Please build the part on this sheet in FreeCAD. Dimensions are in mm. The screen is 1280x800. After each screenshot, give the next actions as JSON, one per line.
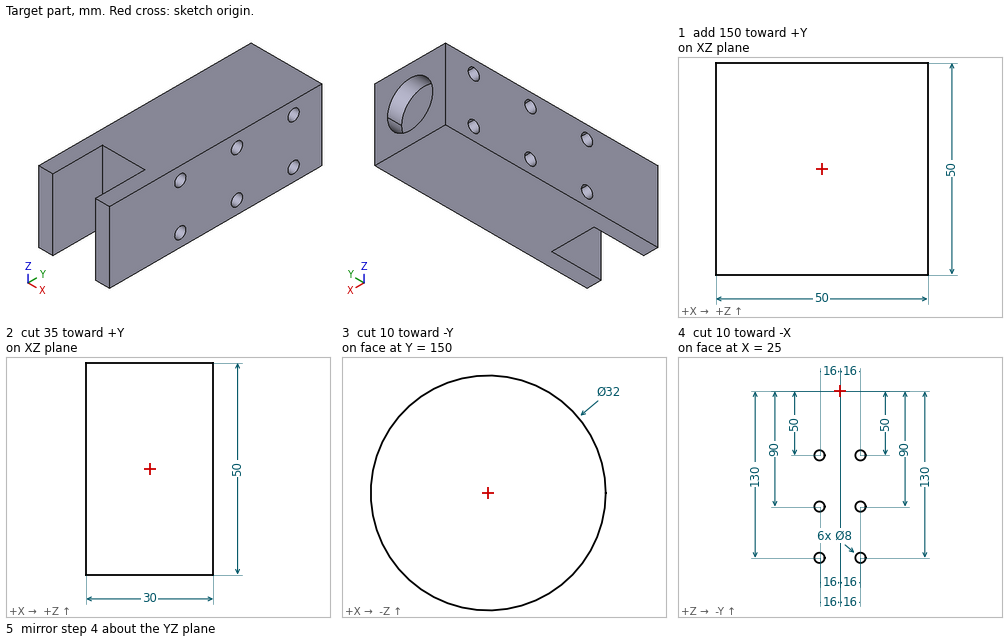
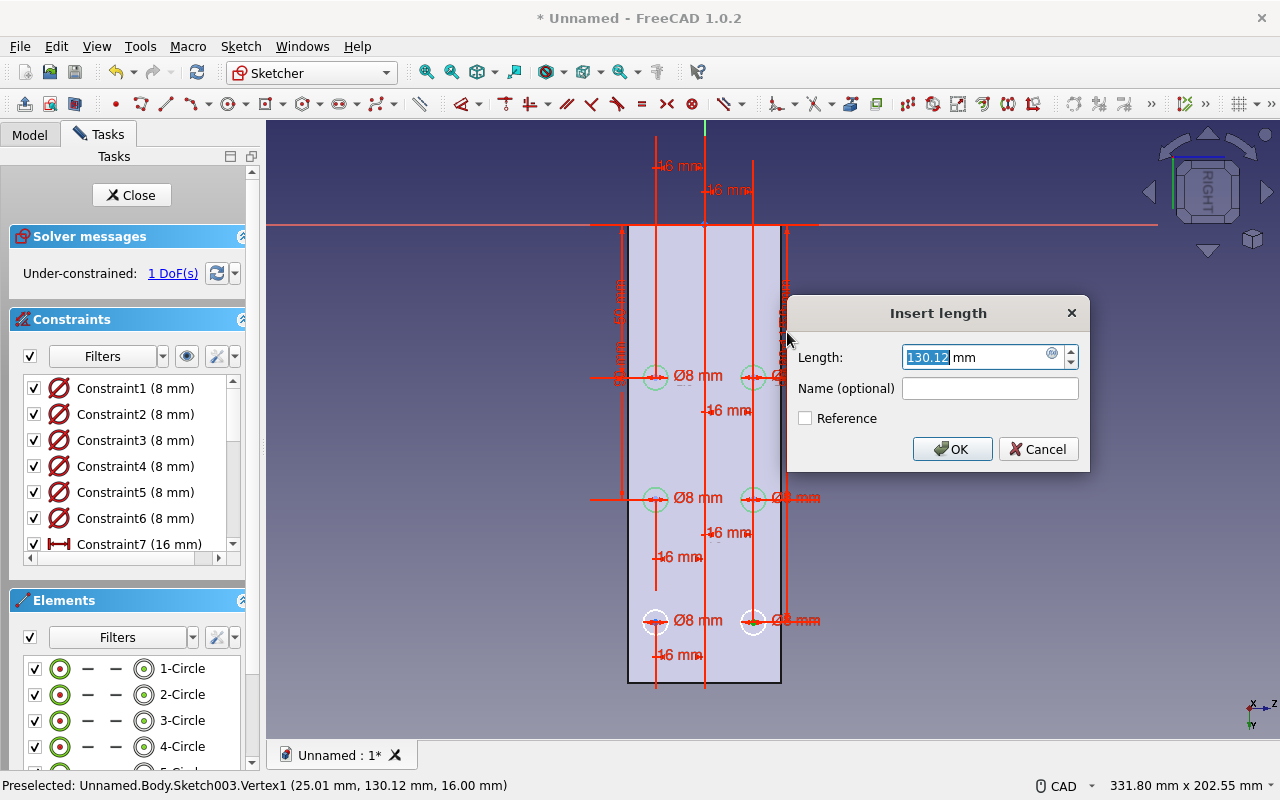
{"action": "type", "text": "130"}
{"action": "key", "text": "Return"}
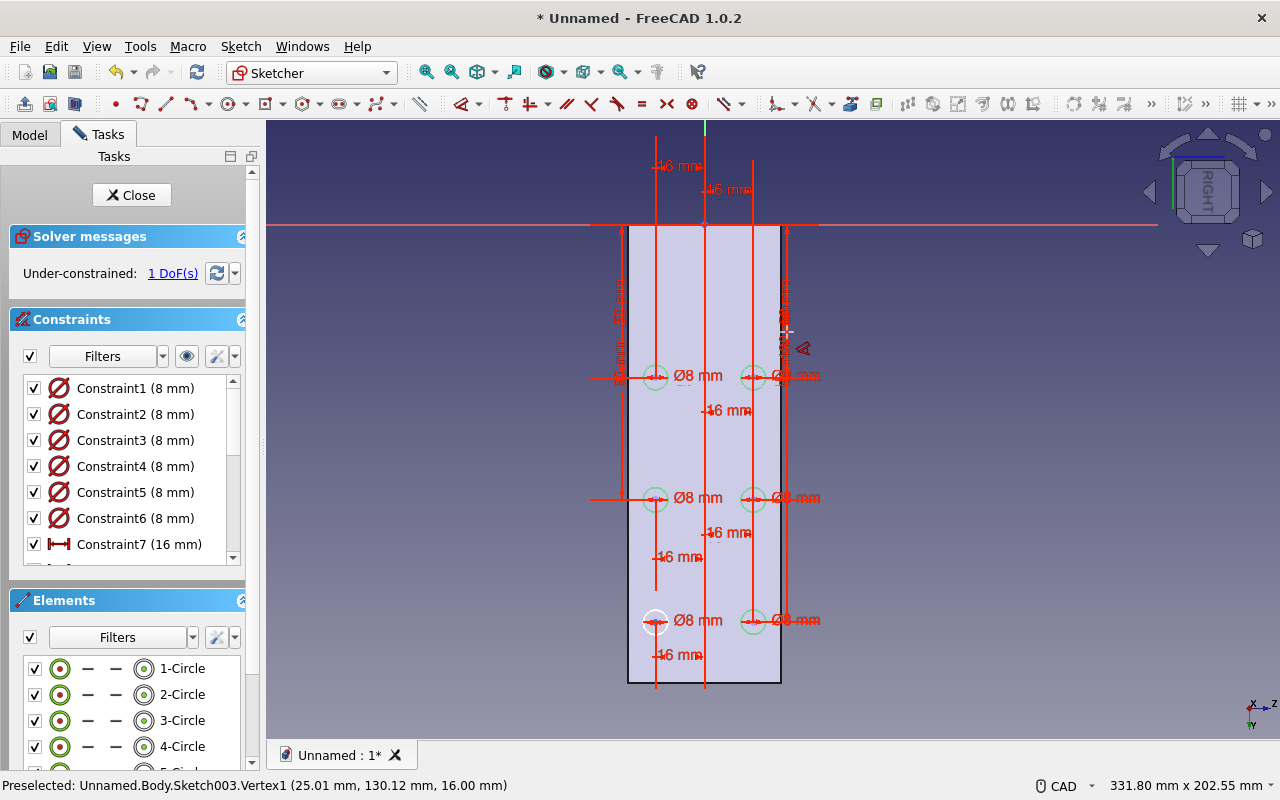
{"action": "left_click", "coordinate": [656, 622]}
{"action": "left_click", "coordinate": [622, 424]}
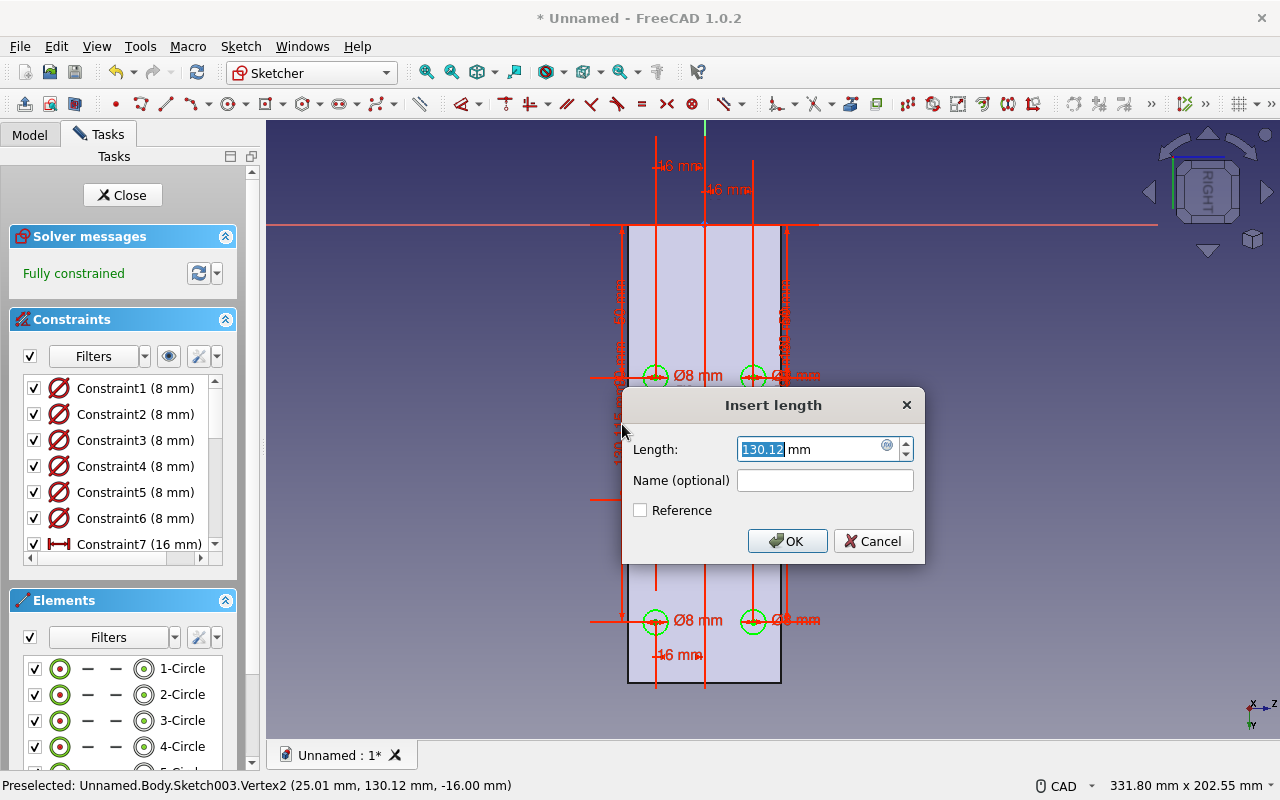
{"action": "type", "text": "130"}
{"action": "key", "text": "Return"}
{"action": "key", "text": "Escape"}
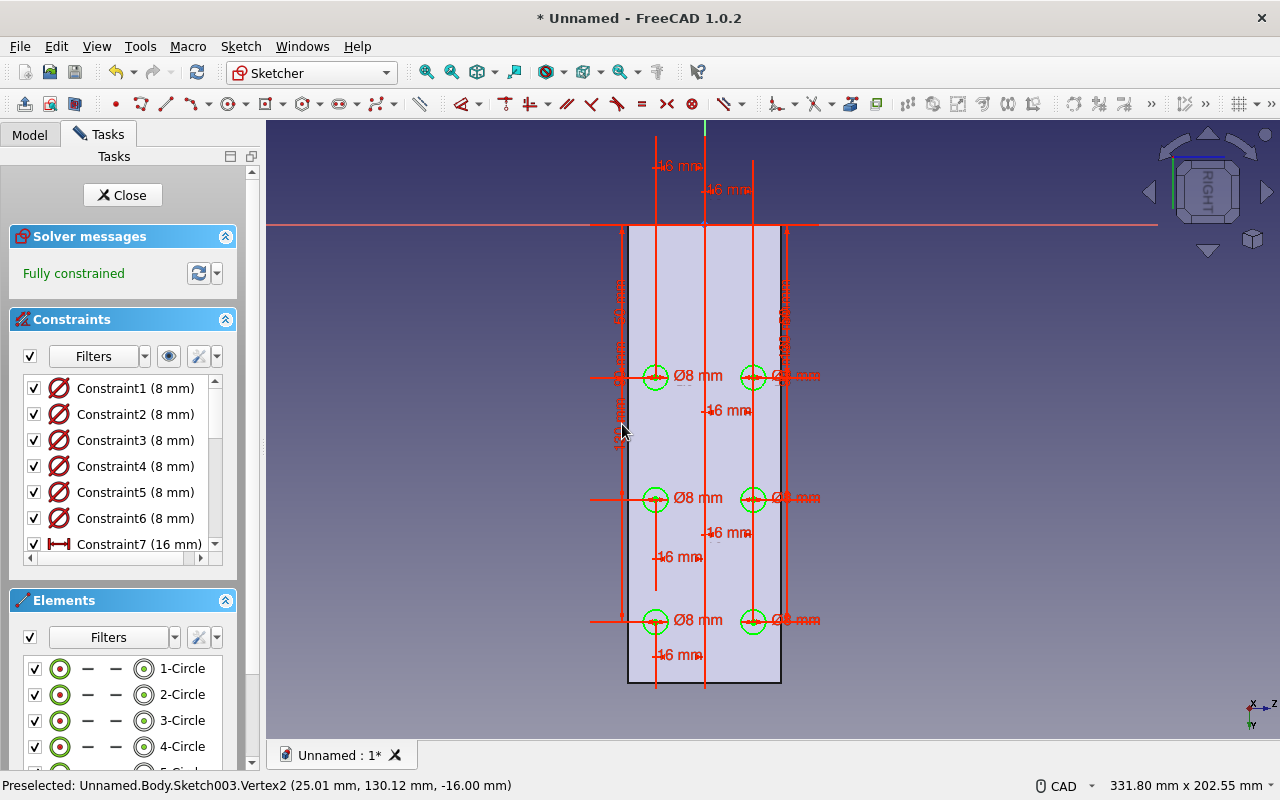
{"action": "left_click", "coordinate": [123, 195]}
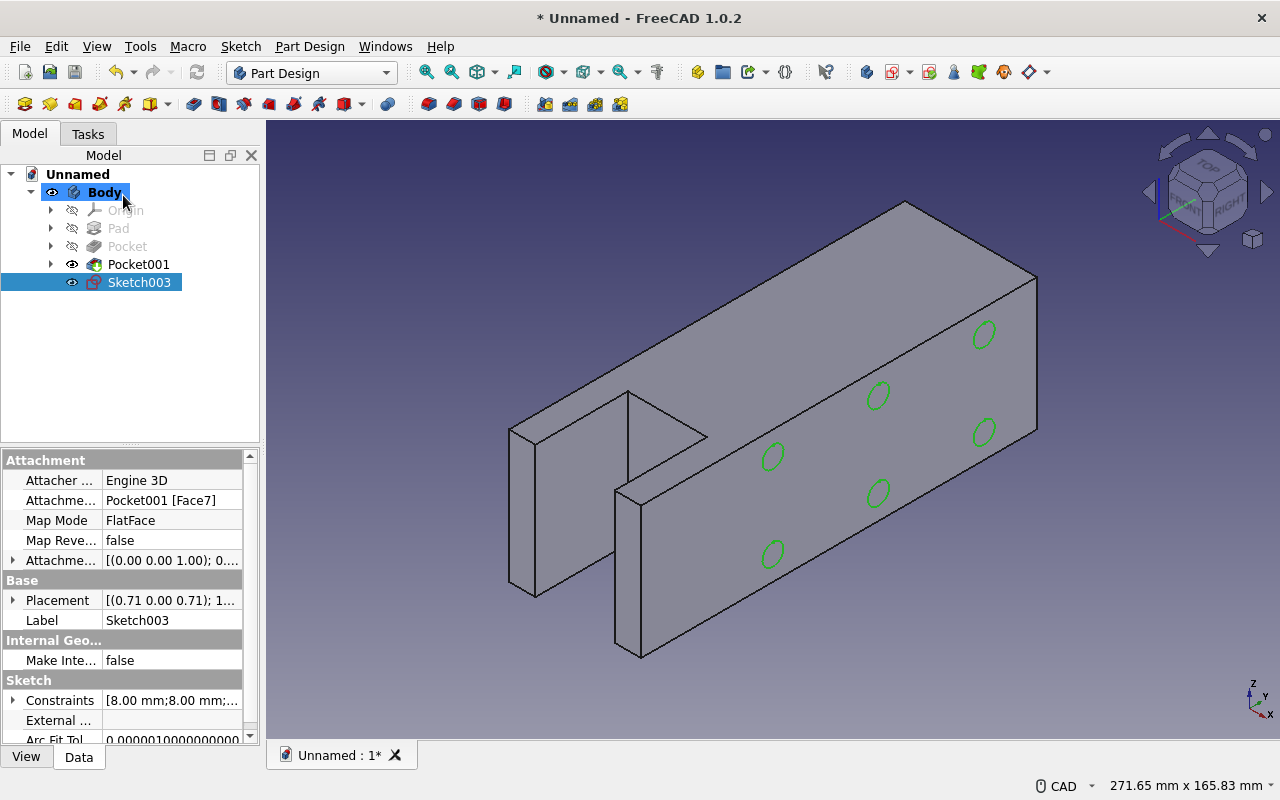
{"action": "left_click", "coordinate": [194, 104]}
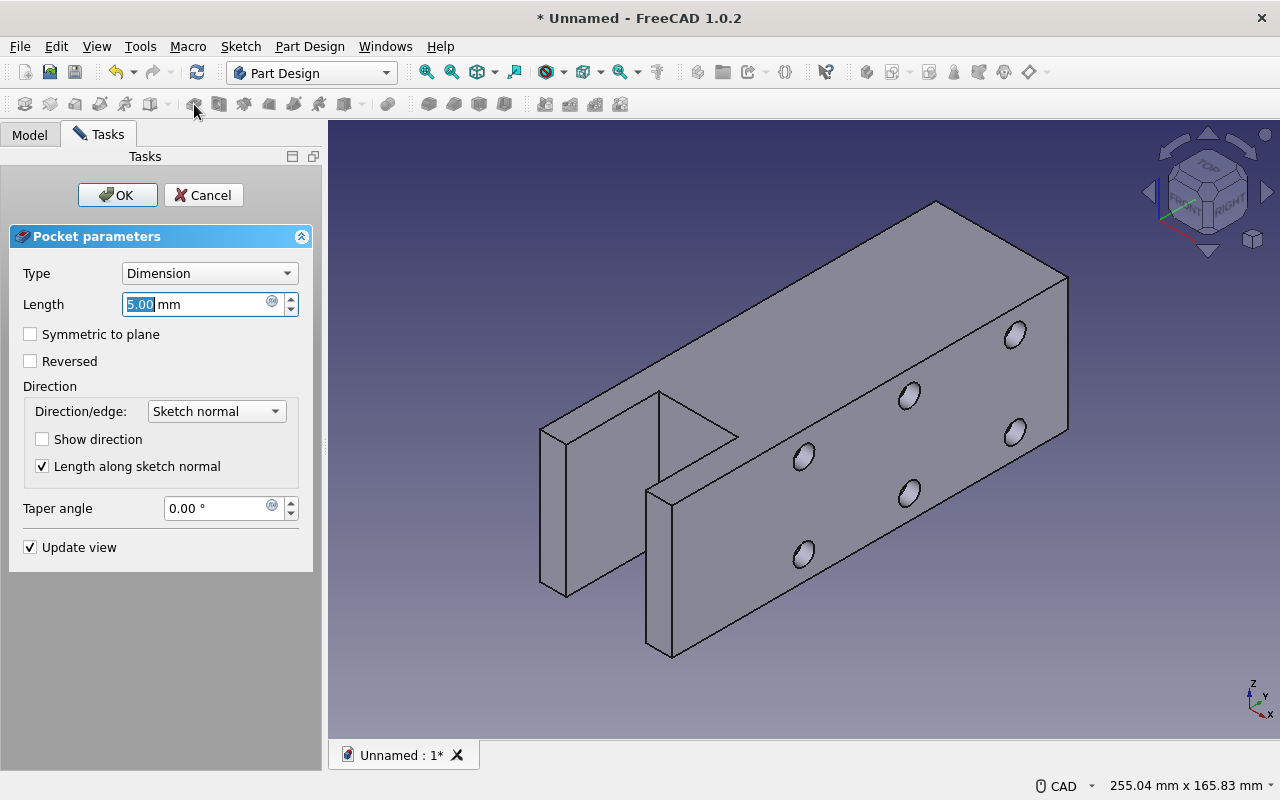
{"action": "type", "text": "10"}
{"action": "key", "text": "Tab"}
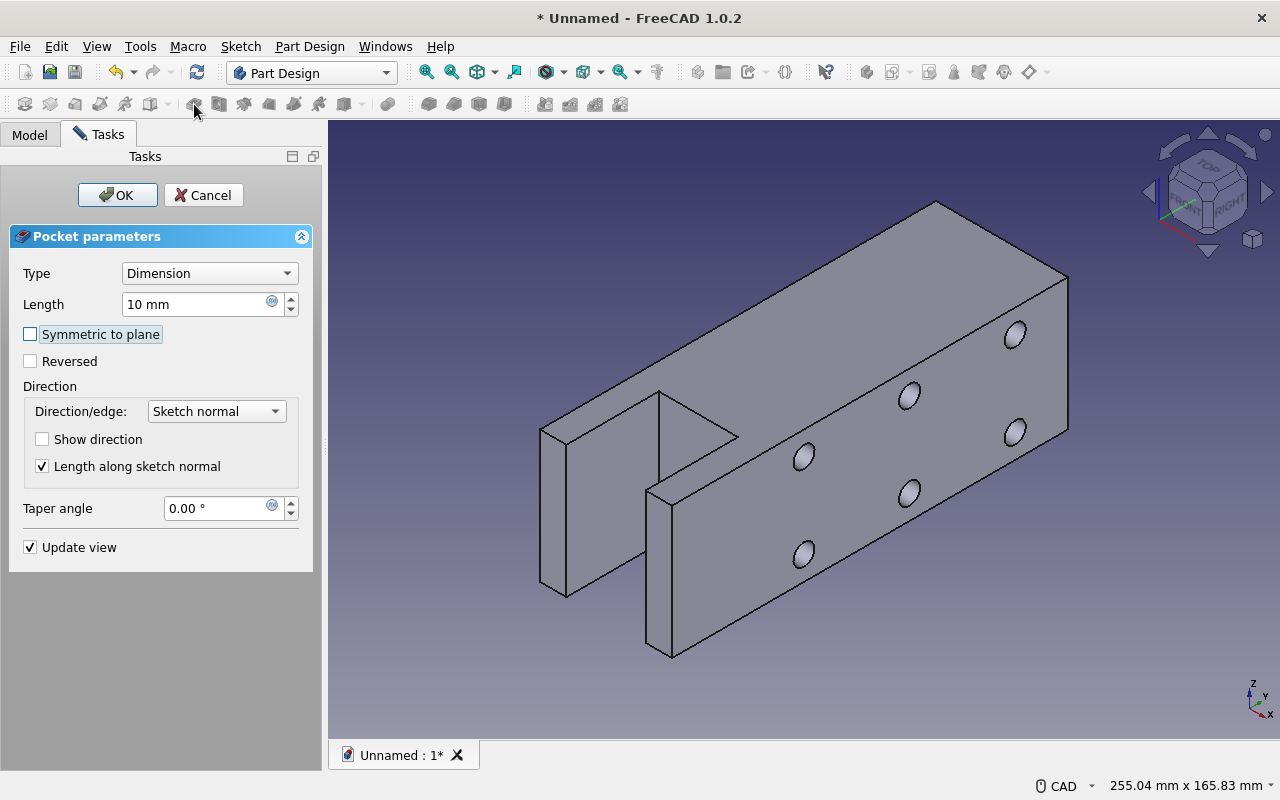
{"action": "left_click", "coordinate": [118, 195]}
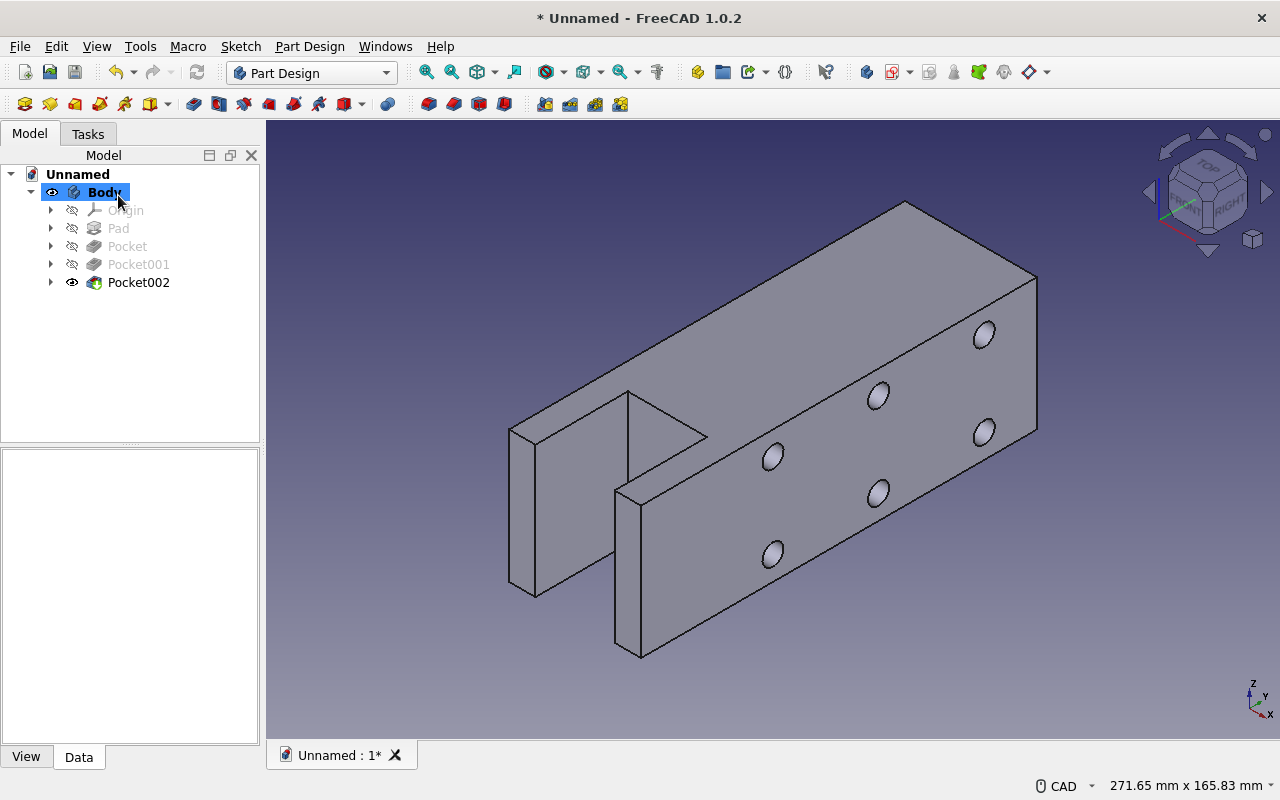
{"action": "left_click", "coordinate": [117, 282]}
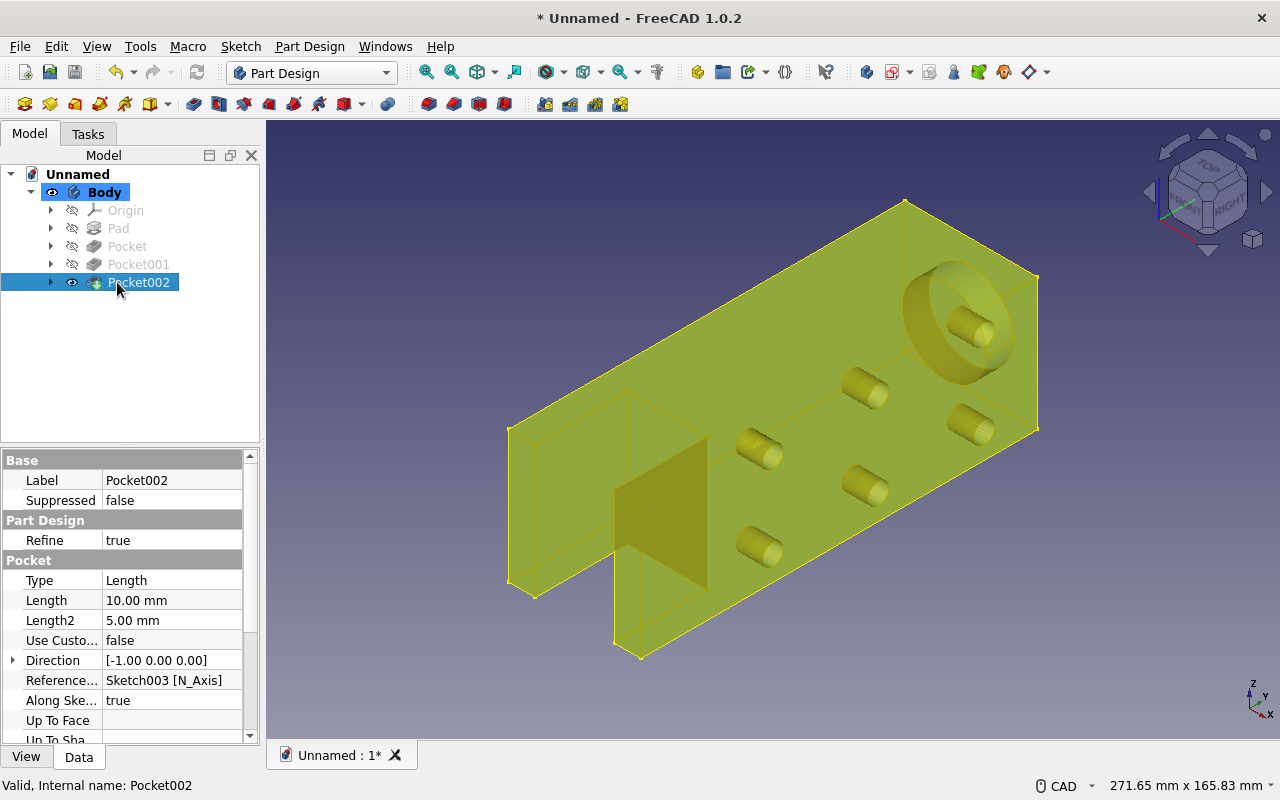
{"action": "left_click", "coordinate": [545, 104]}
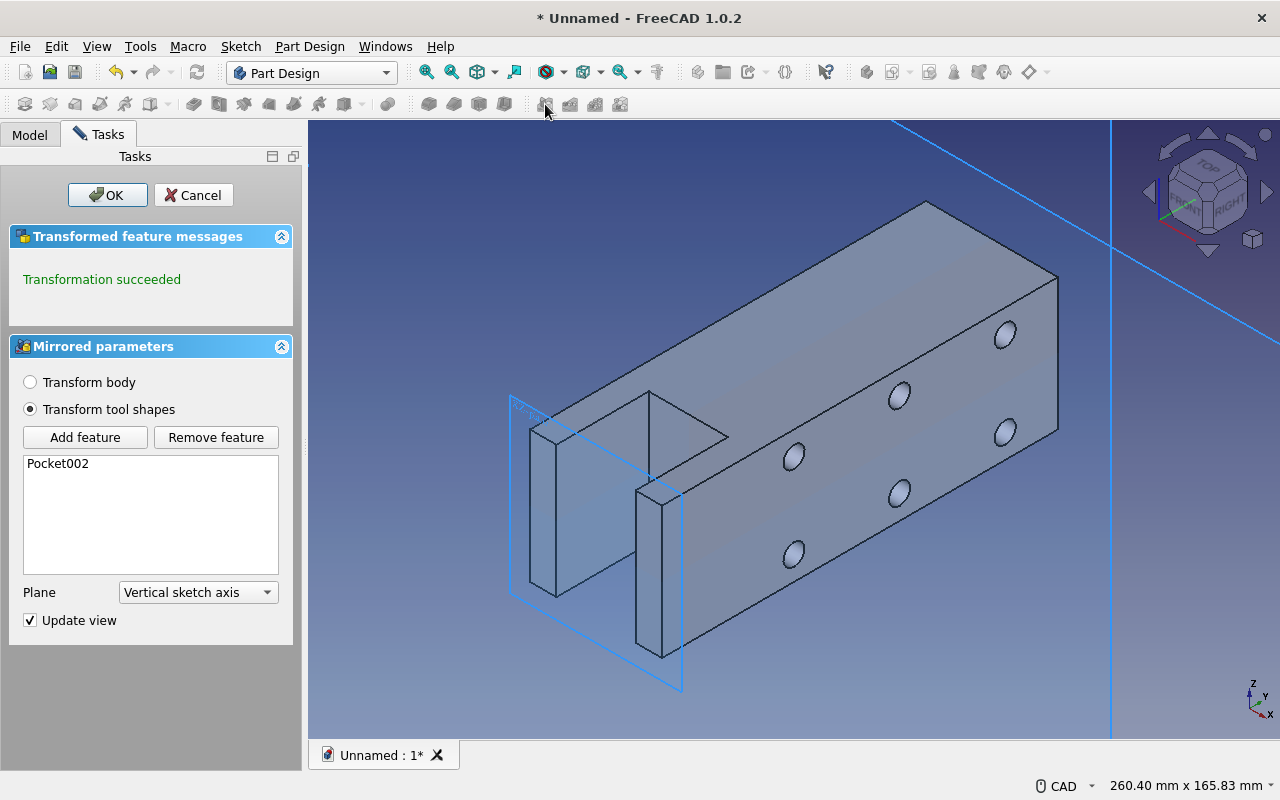
{"action": "left_click", "coordinate": [199, 592]}